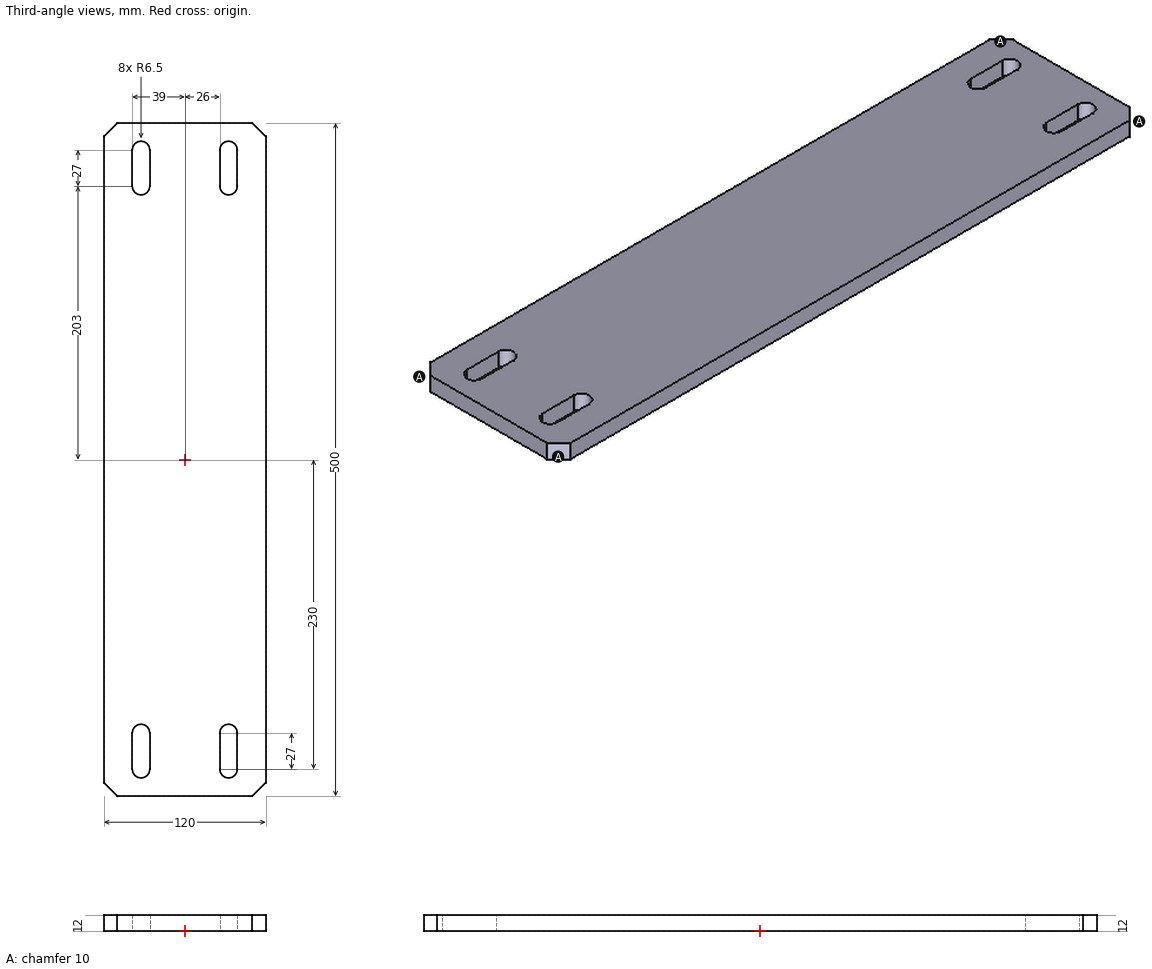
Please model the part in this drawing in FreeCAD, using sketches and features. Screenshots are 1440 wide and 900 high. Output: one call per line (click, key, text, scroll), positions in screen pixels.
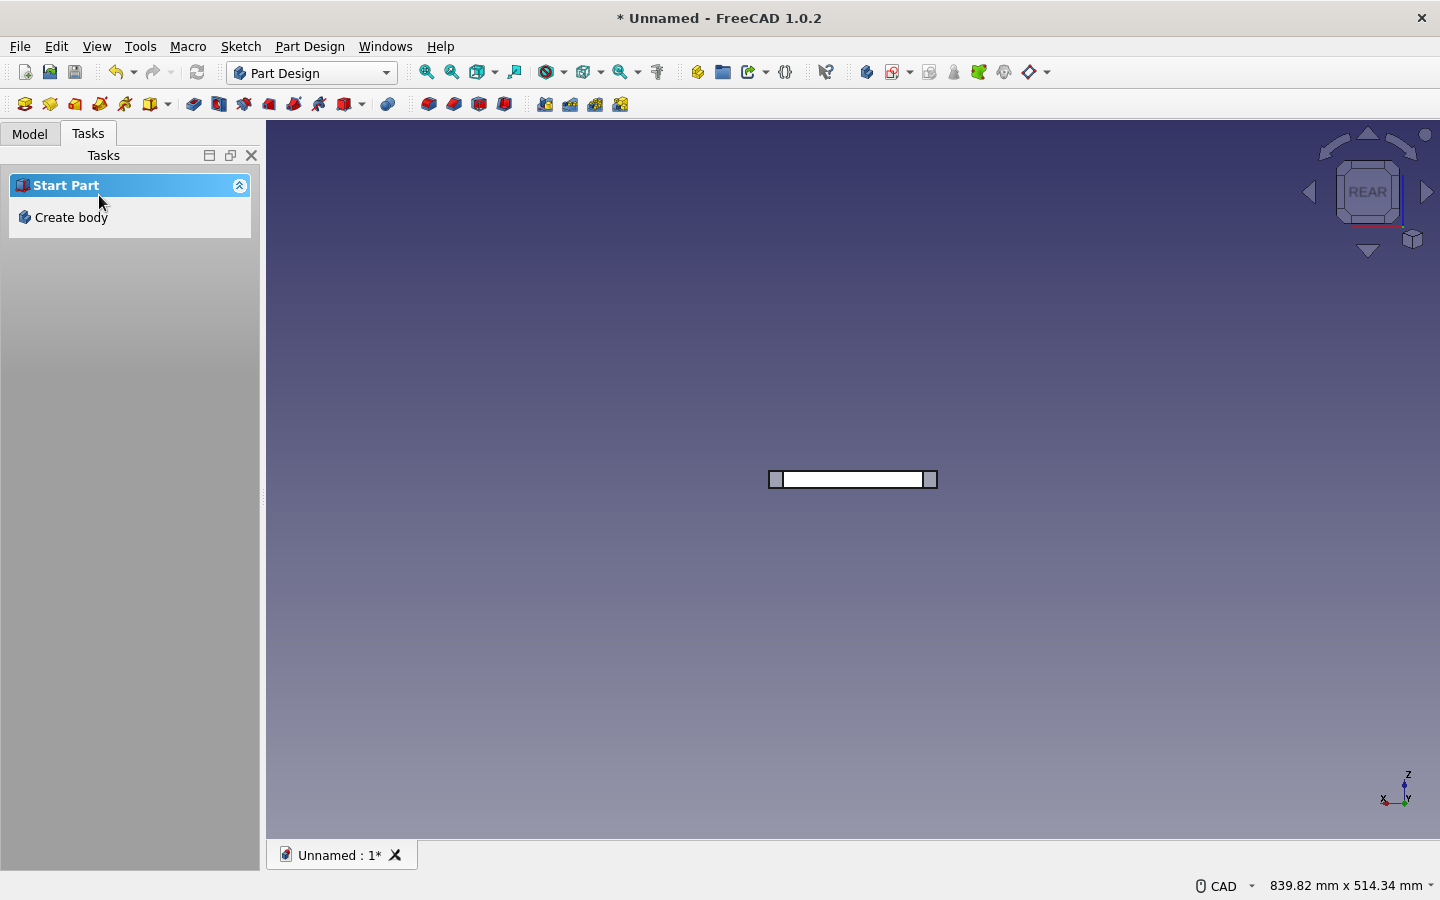
key(0)